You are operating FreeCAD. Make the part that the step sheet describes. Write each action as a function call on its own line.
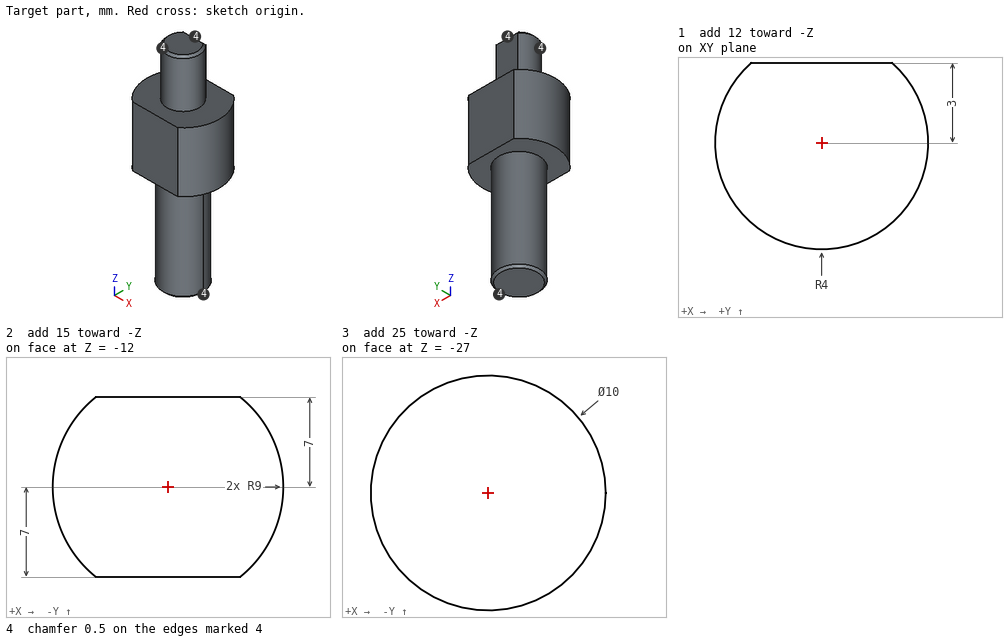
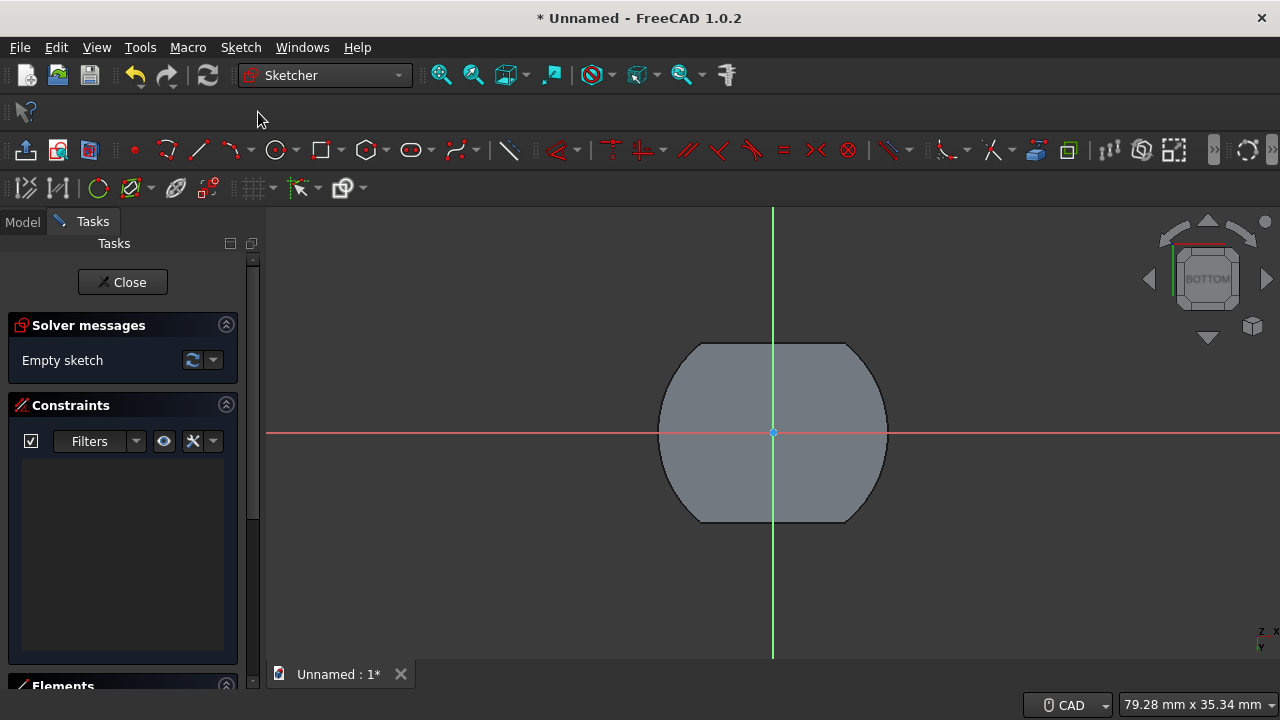
scroll(829, 433, up, 4)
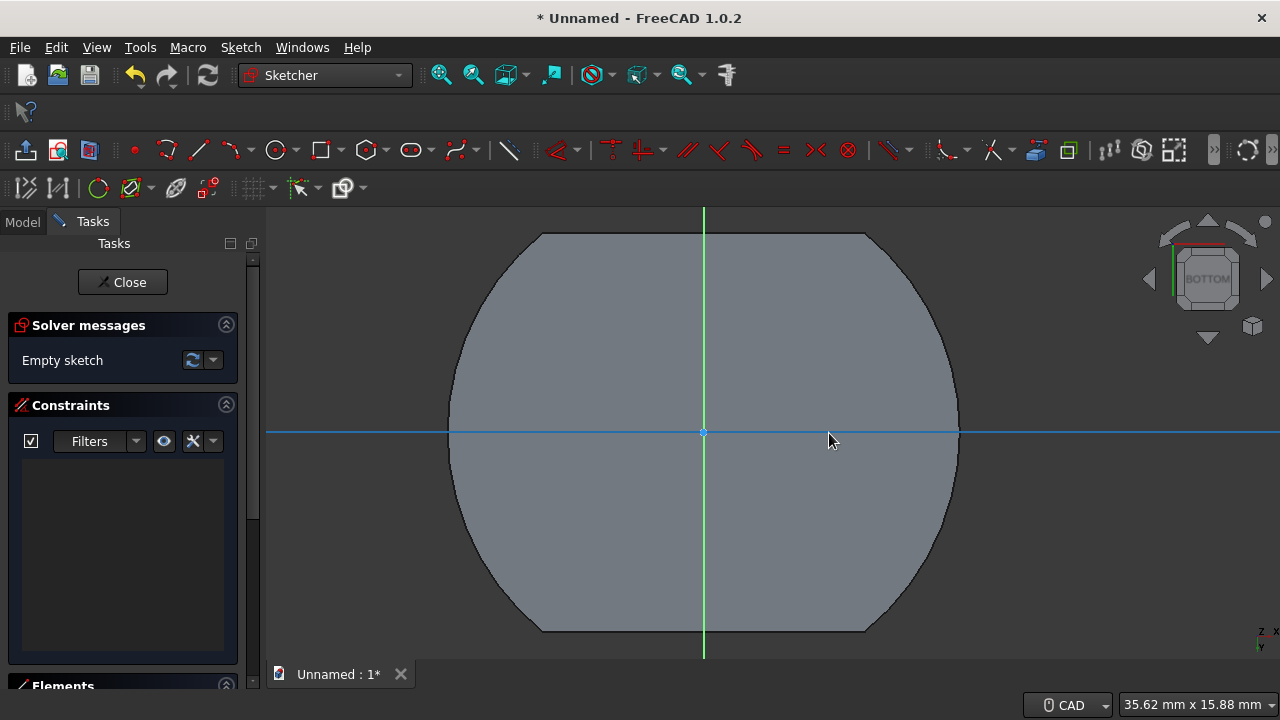
key(g)
key(c)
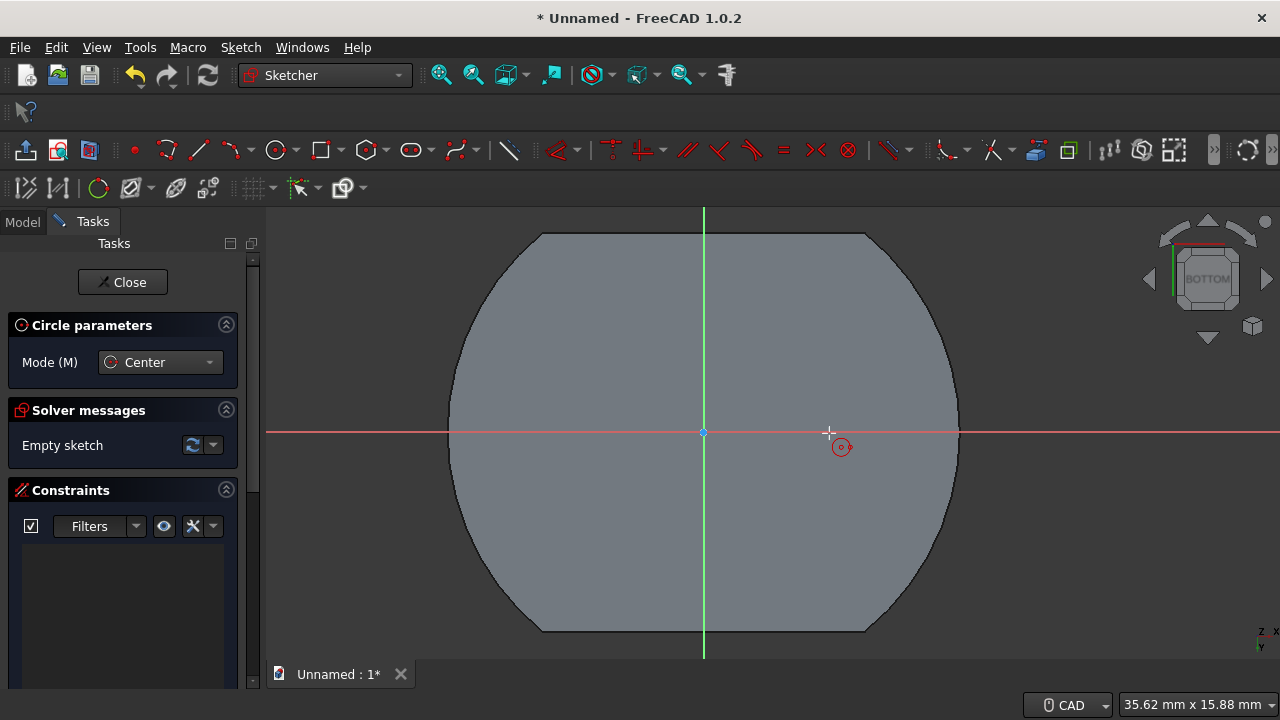
click(704, 432)
click(804, 332)
key(Escape)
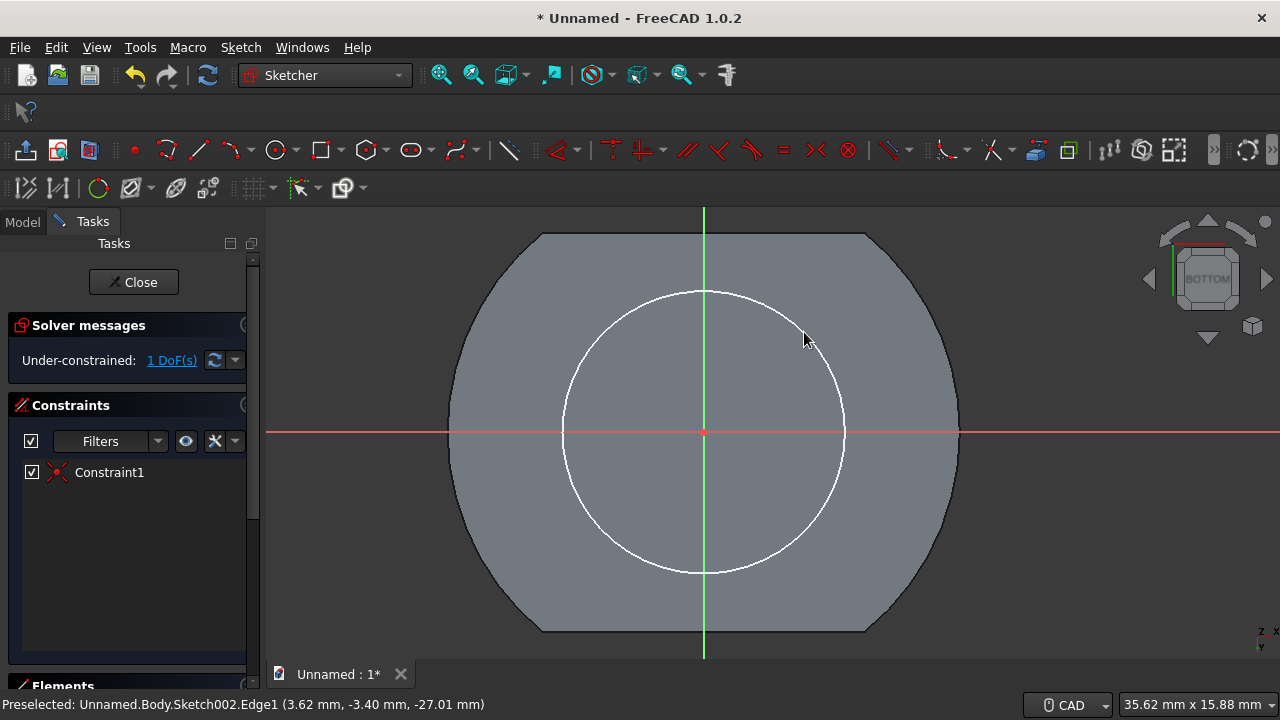
key(d)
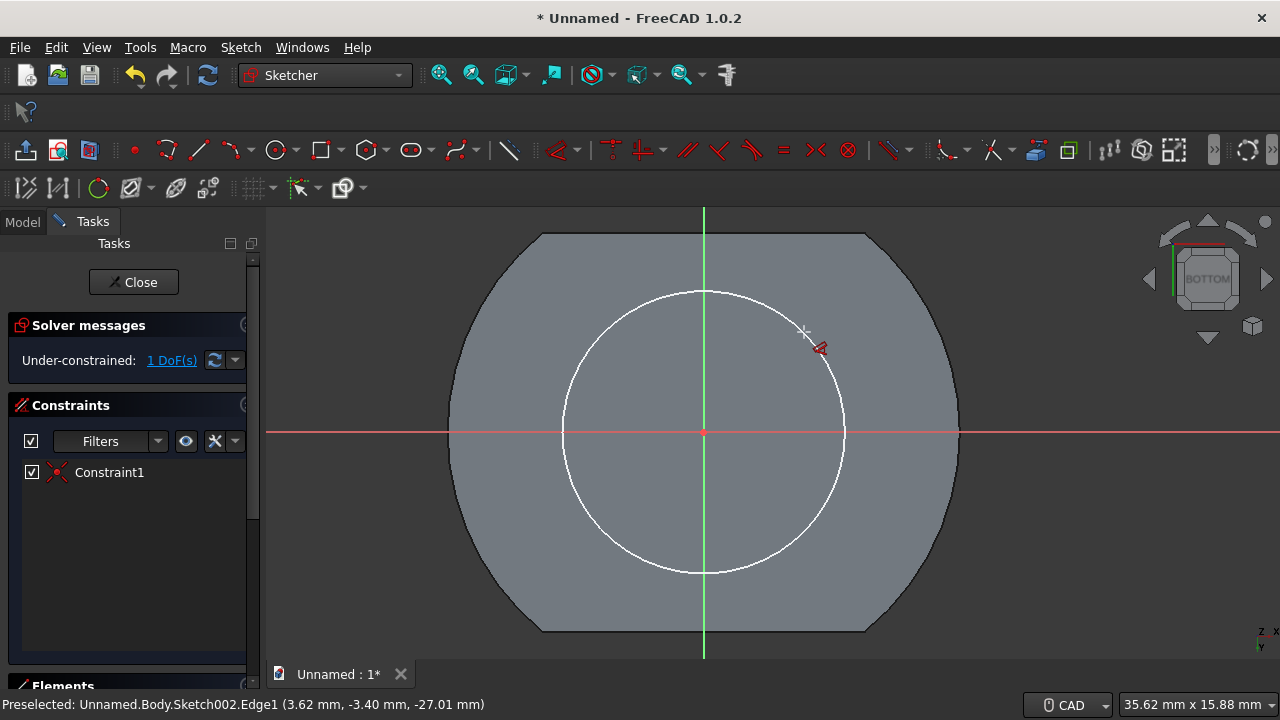
click(803, 332)
click(826, 309)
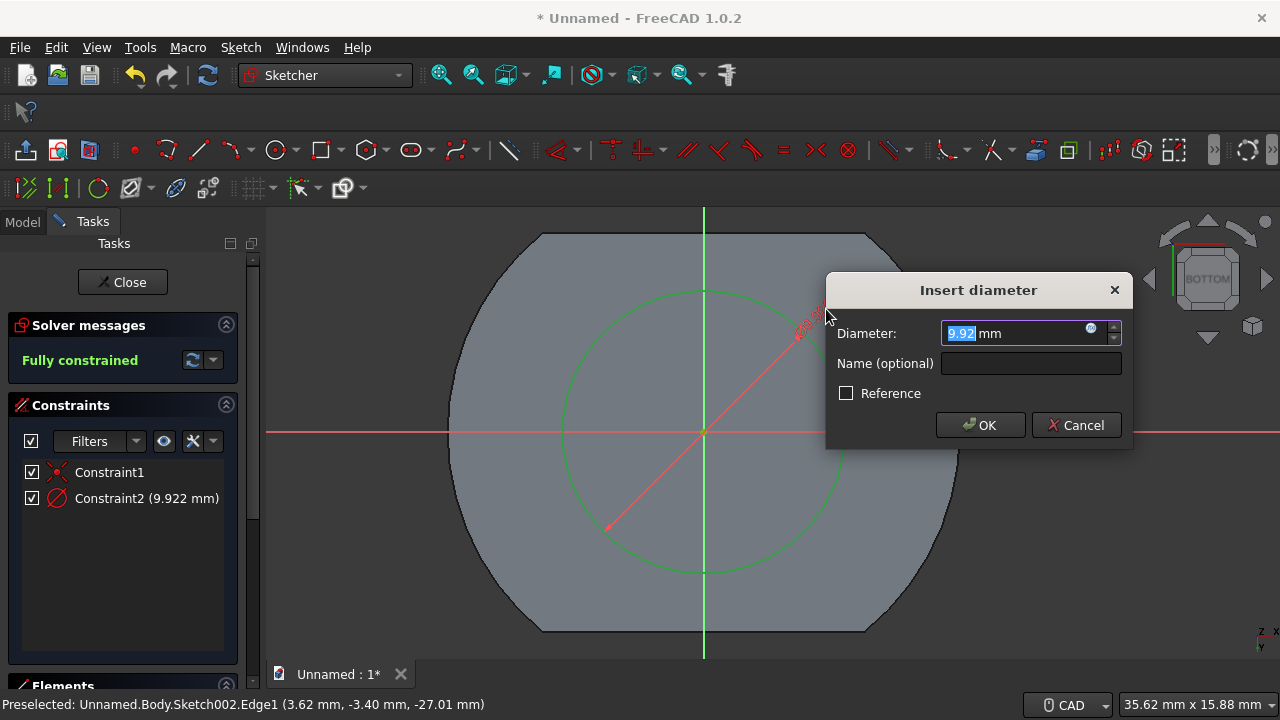
text(10)
key(Return)
key(Escape)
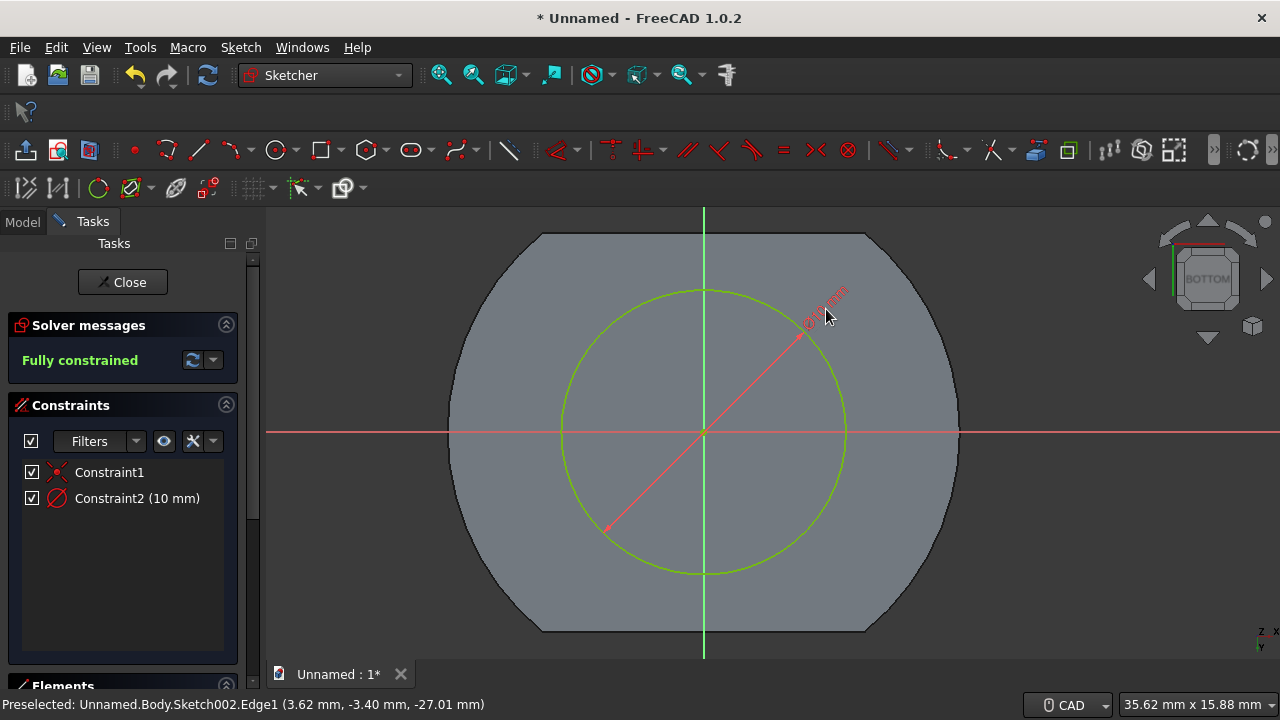
click(123, 282)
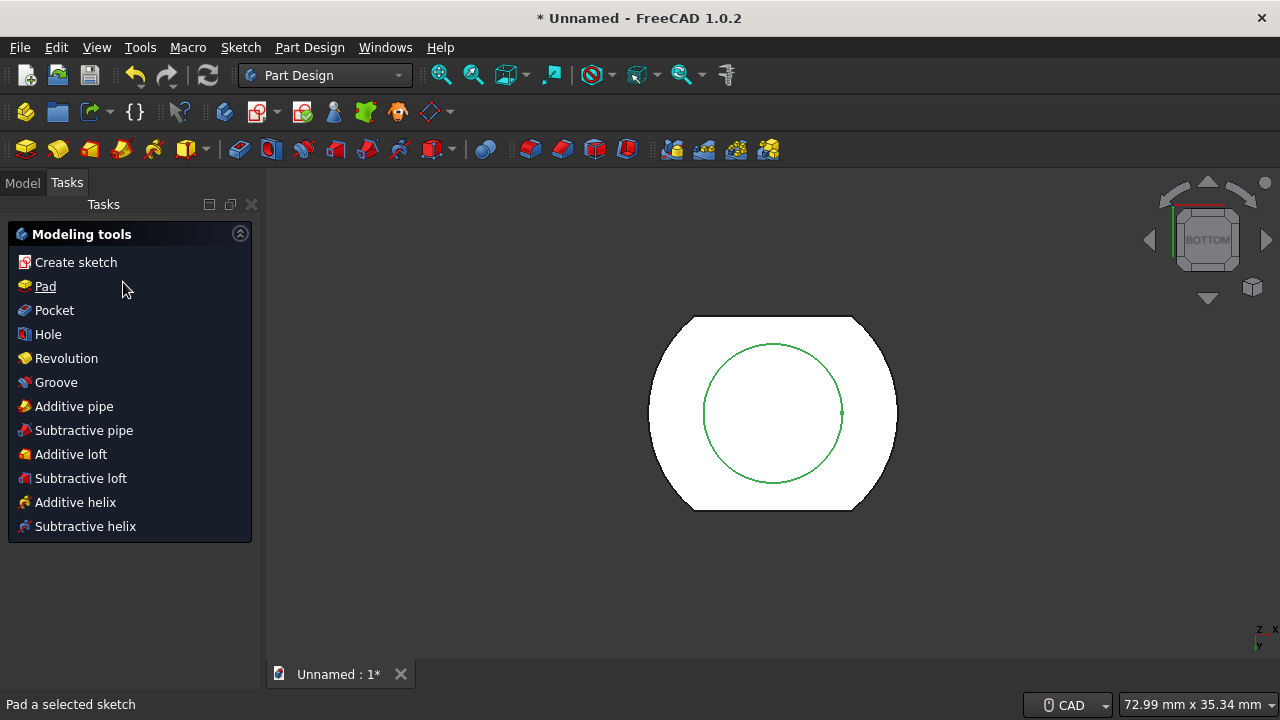
click(26, 150)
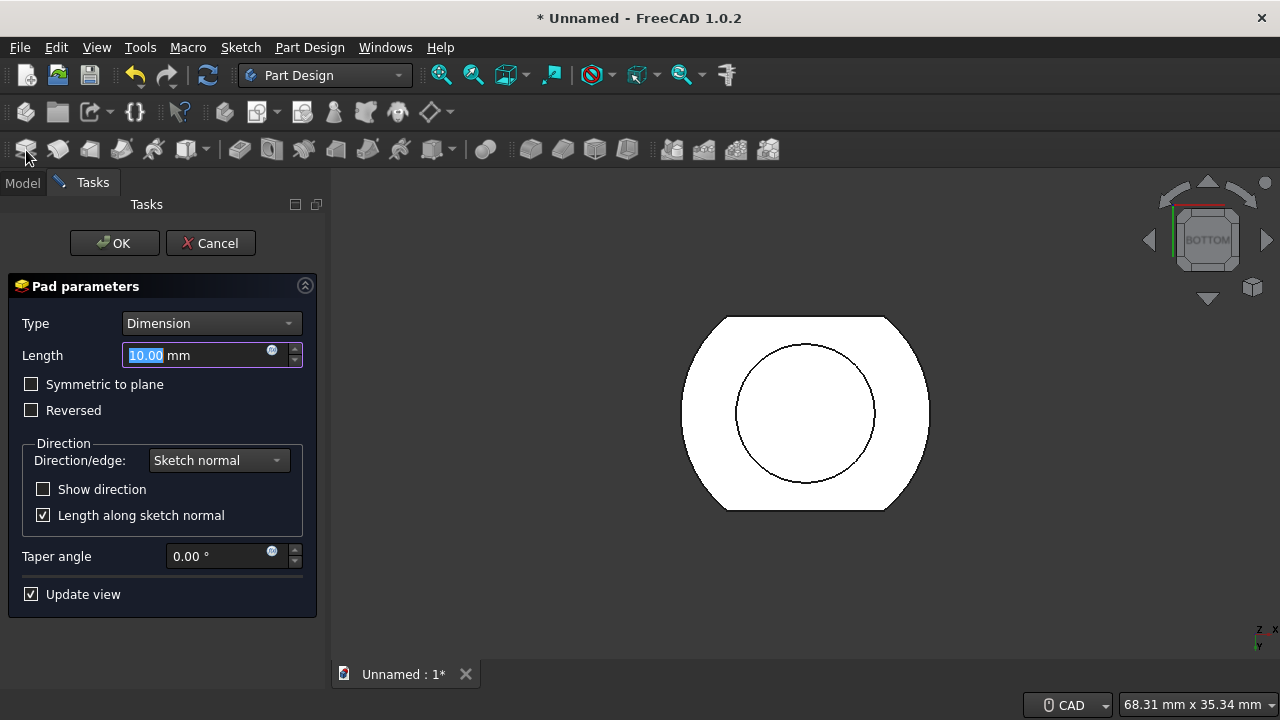
text(25)
key(Tab)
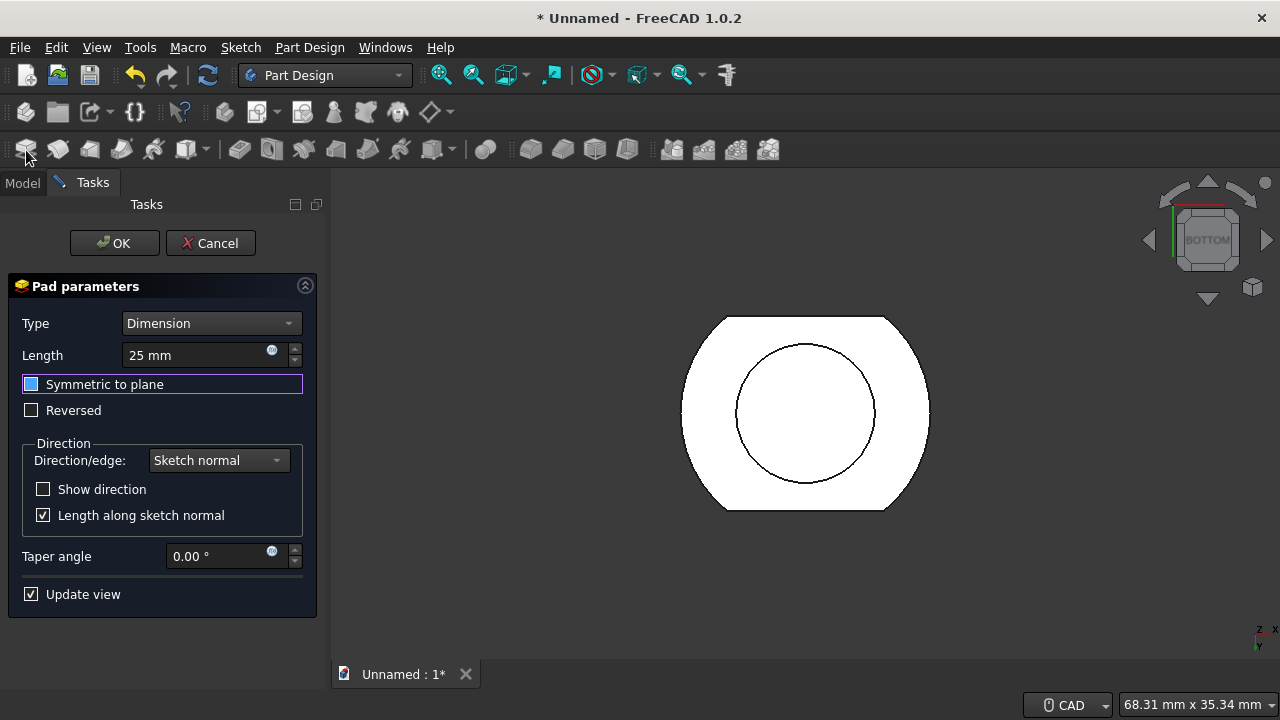
click(115, 243)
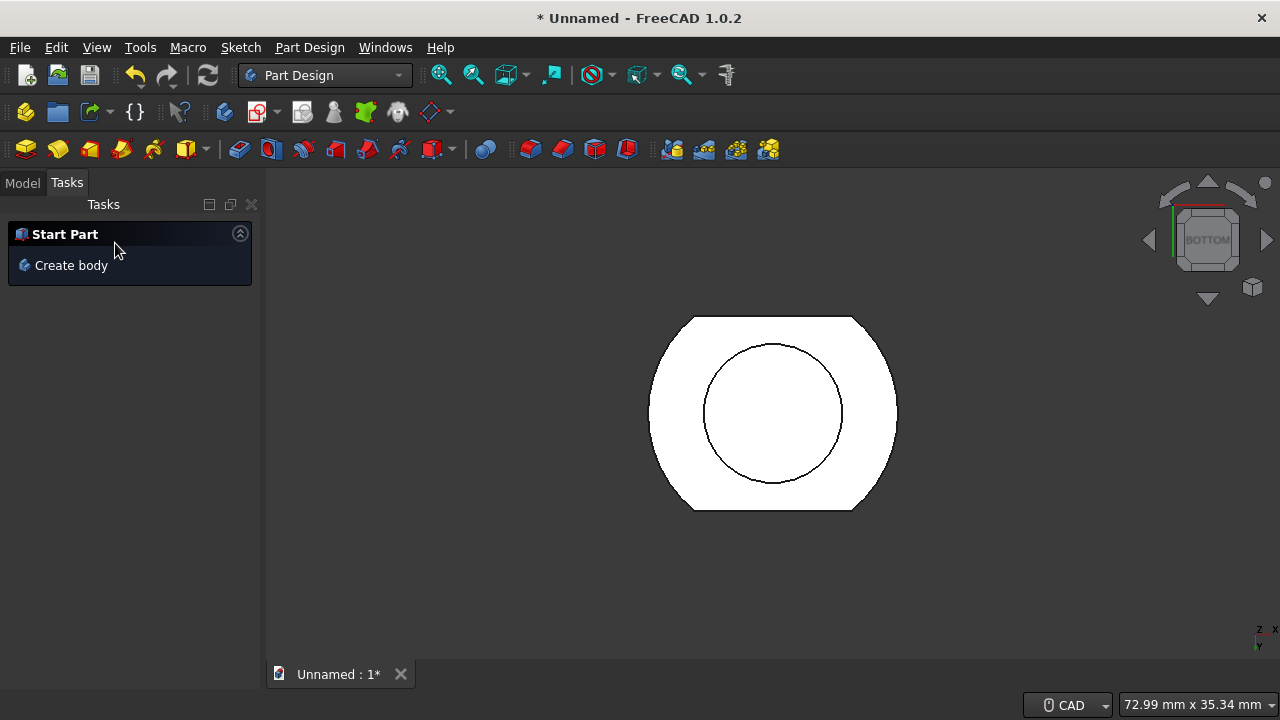
key(v)
key(f)